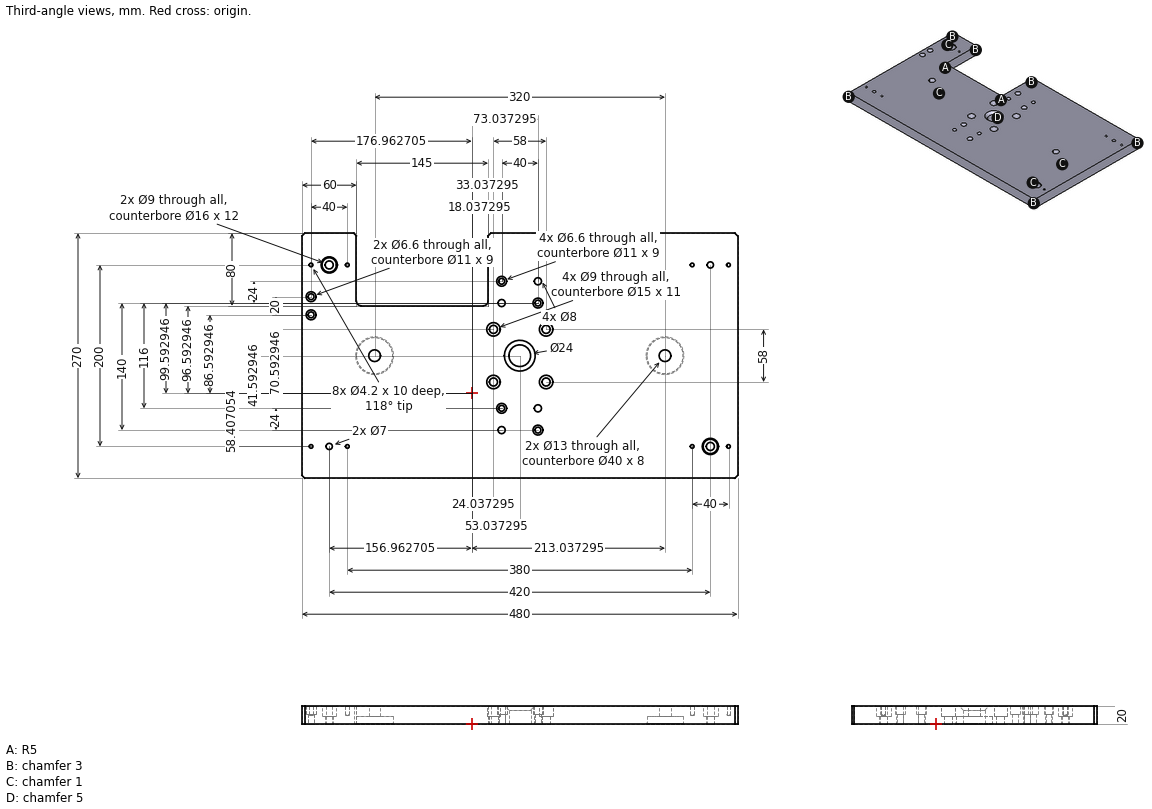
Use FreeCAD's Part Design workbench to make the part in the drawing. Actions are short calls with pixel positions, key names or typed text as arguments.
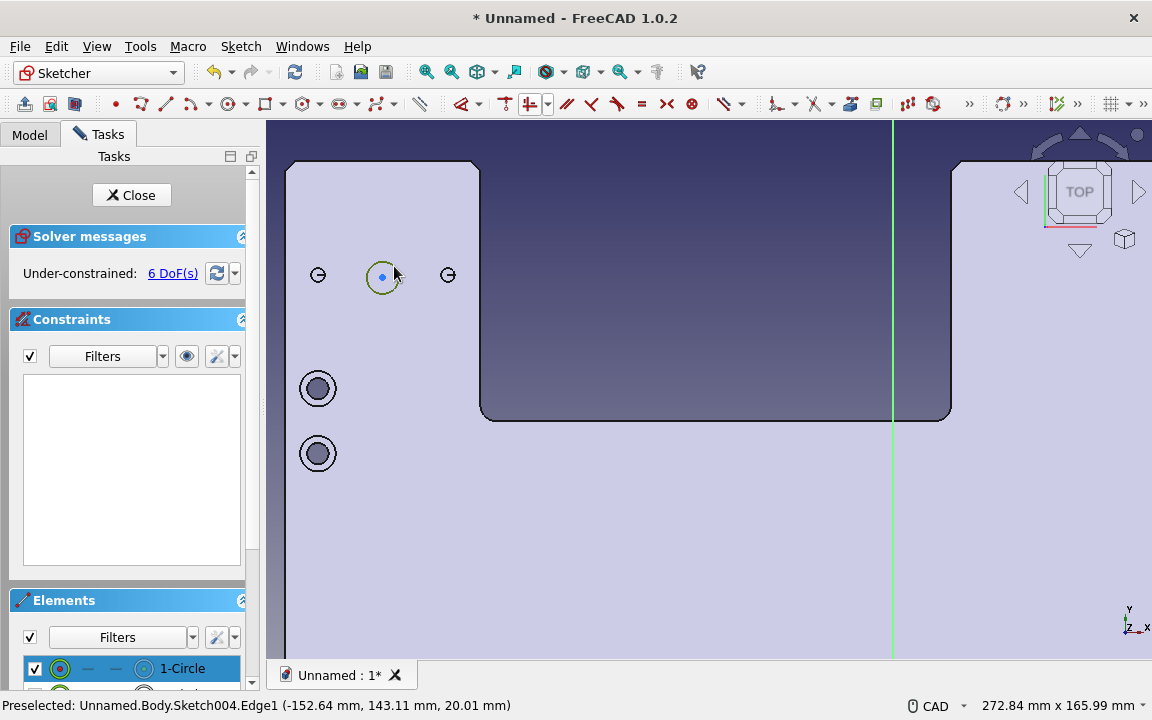
scroll(394, 267, down, 5)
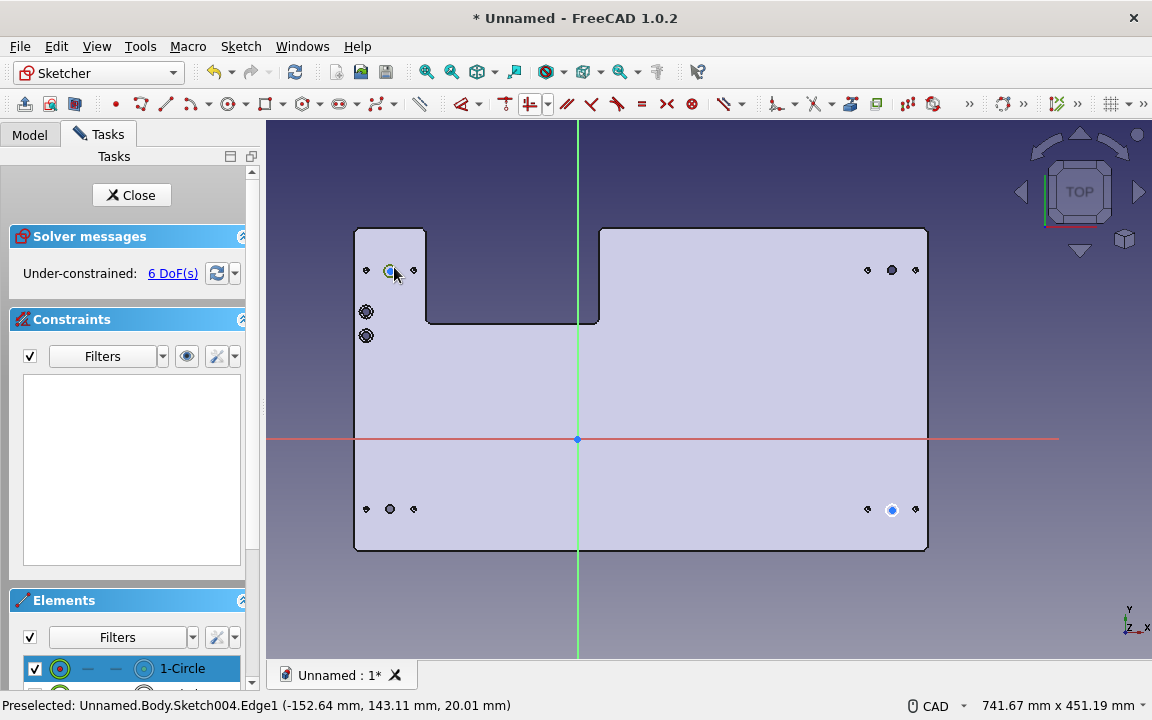
scroll(896, 506, up, 5)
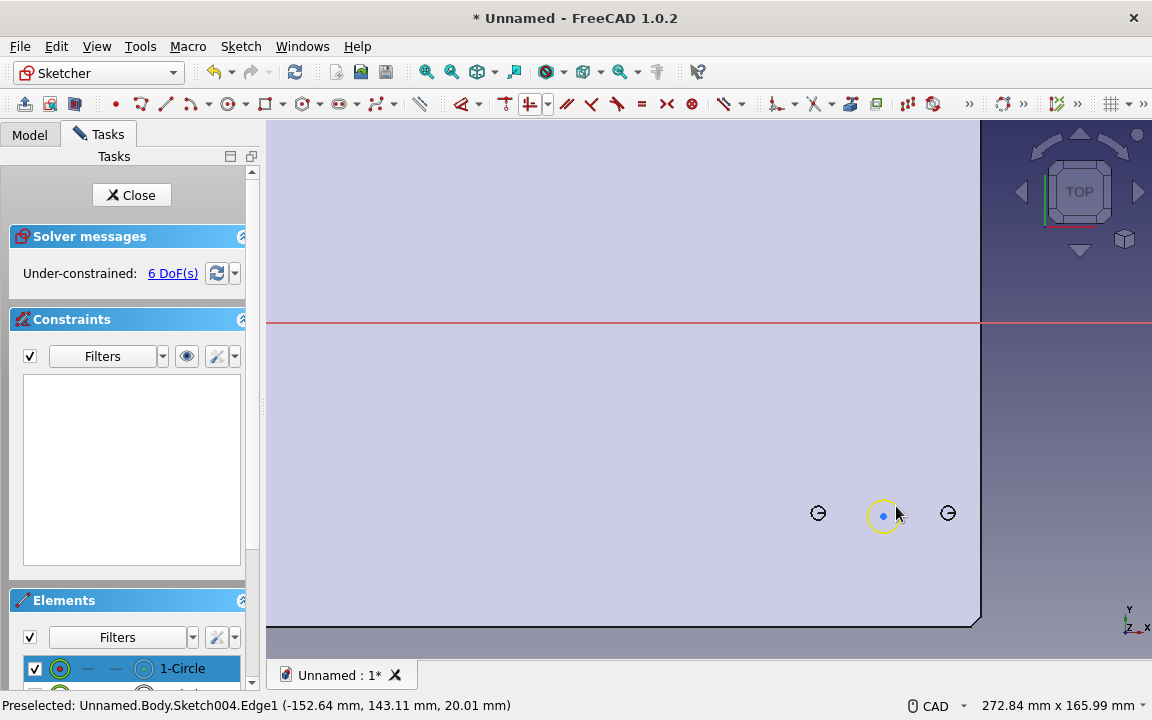
click(895, 505)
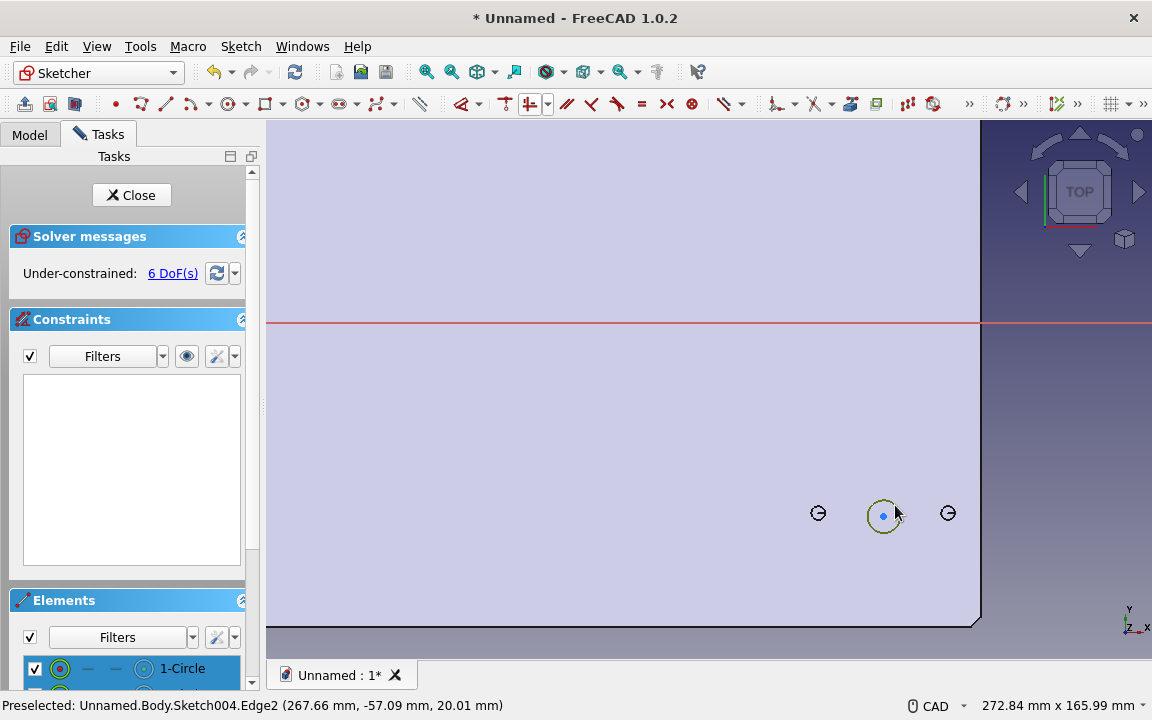
key(e)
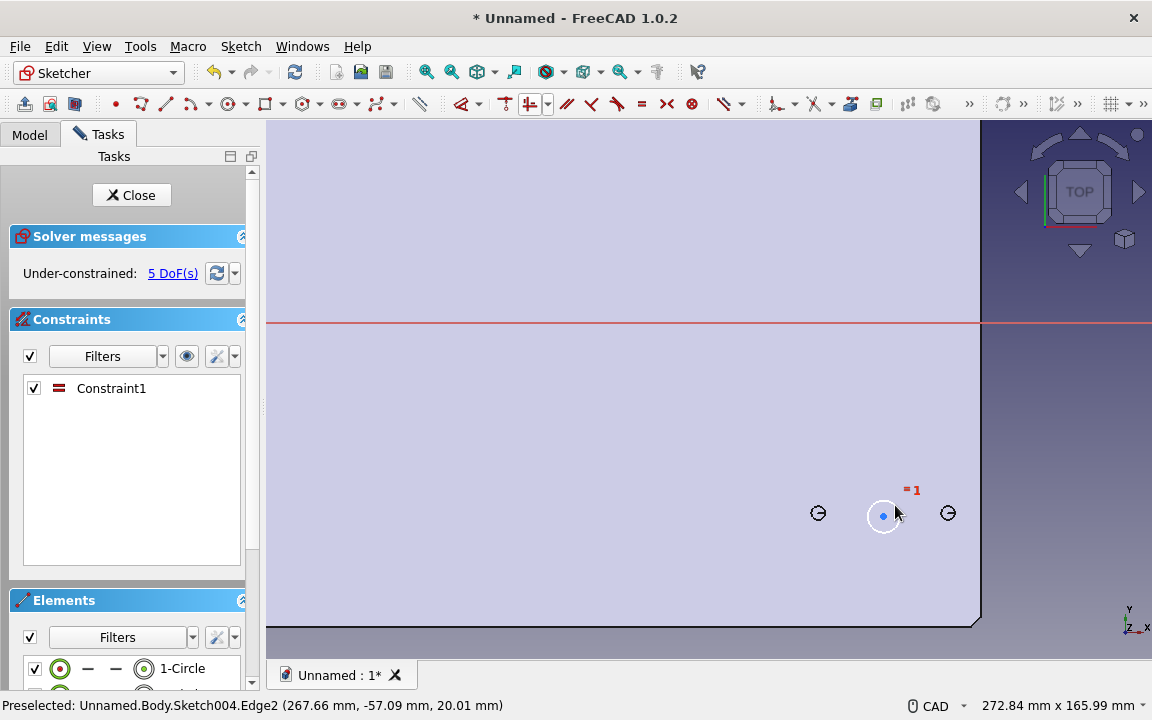
key(d)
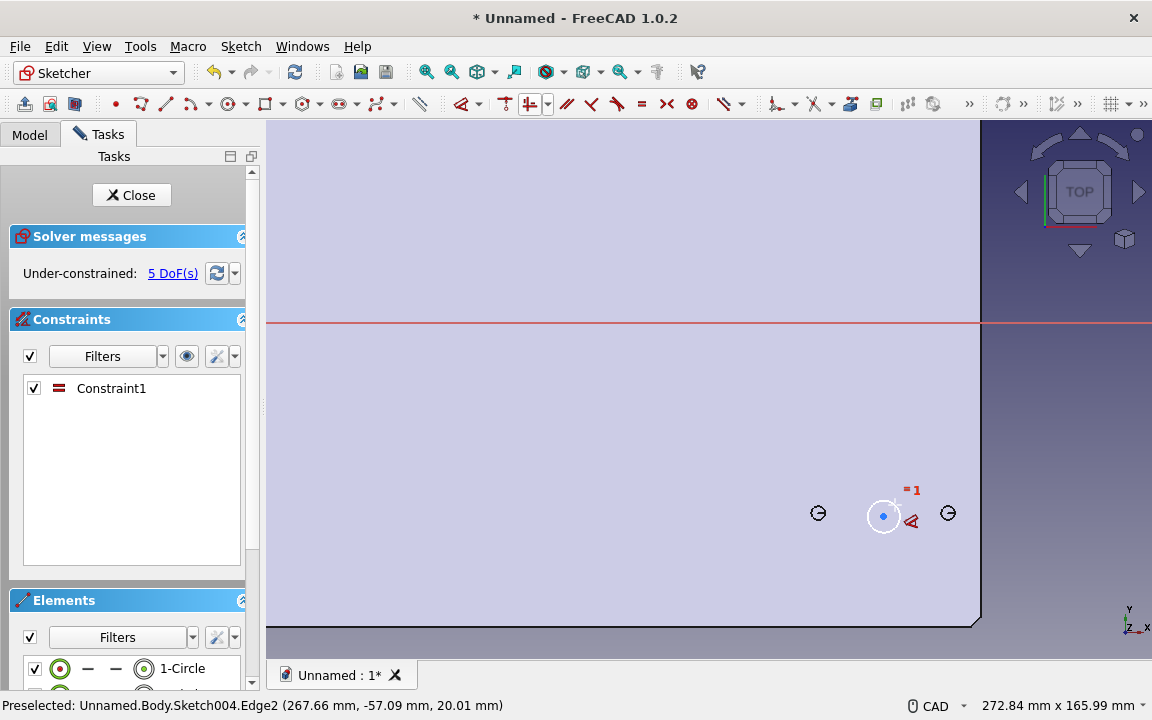
scroll(896, 507, down, 5)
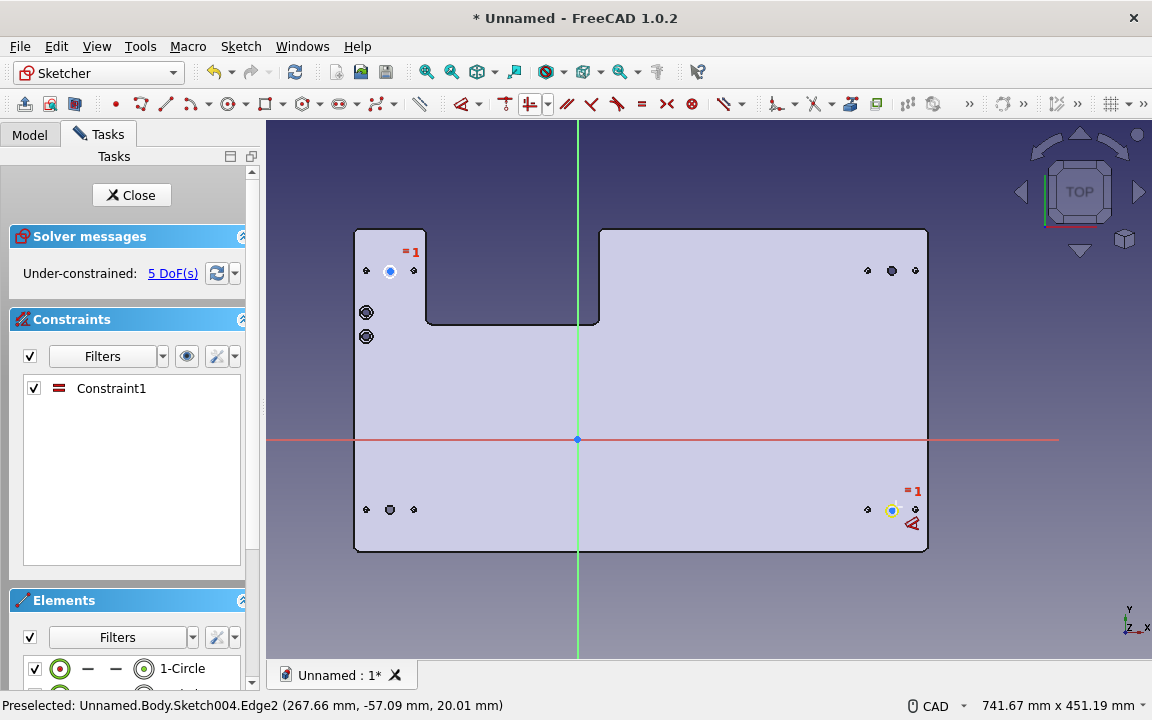
scroll(394, 268, up, 7)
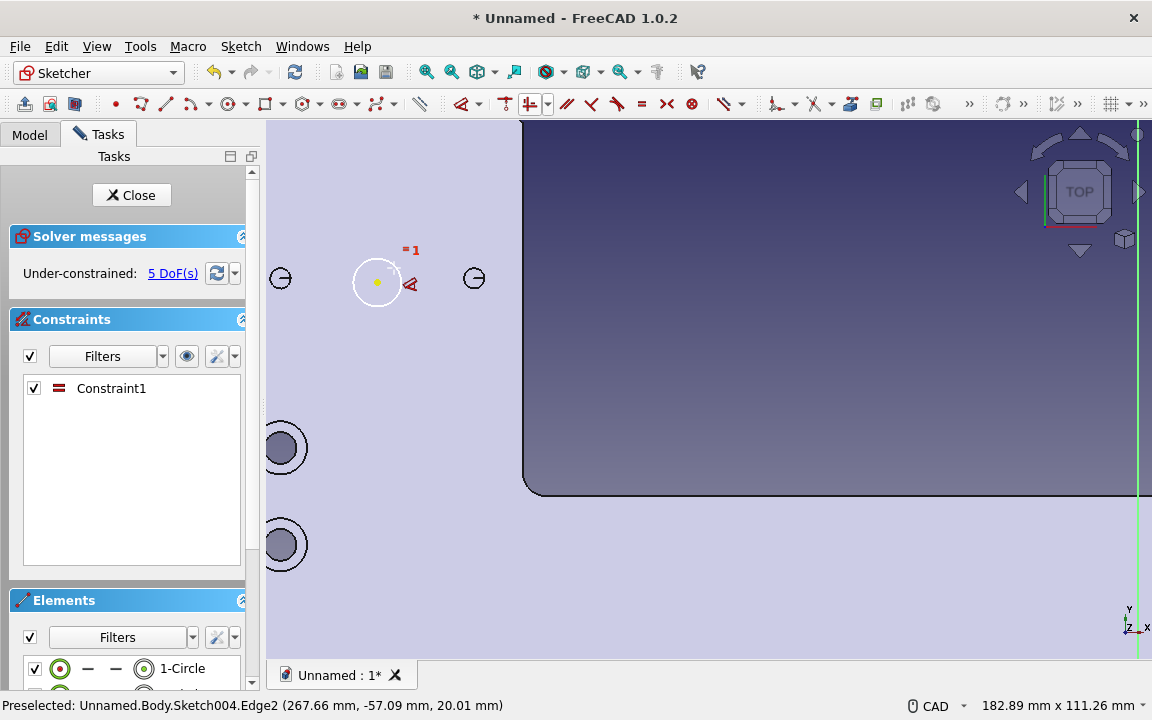
click(394, 266)
click(417, 243)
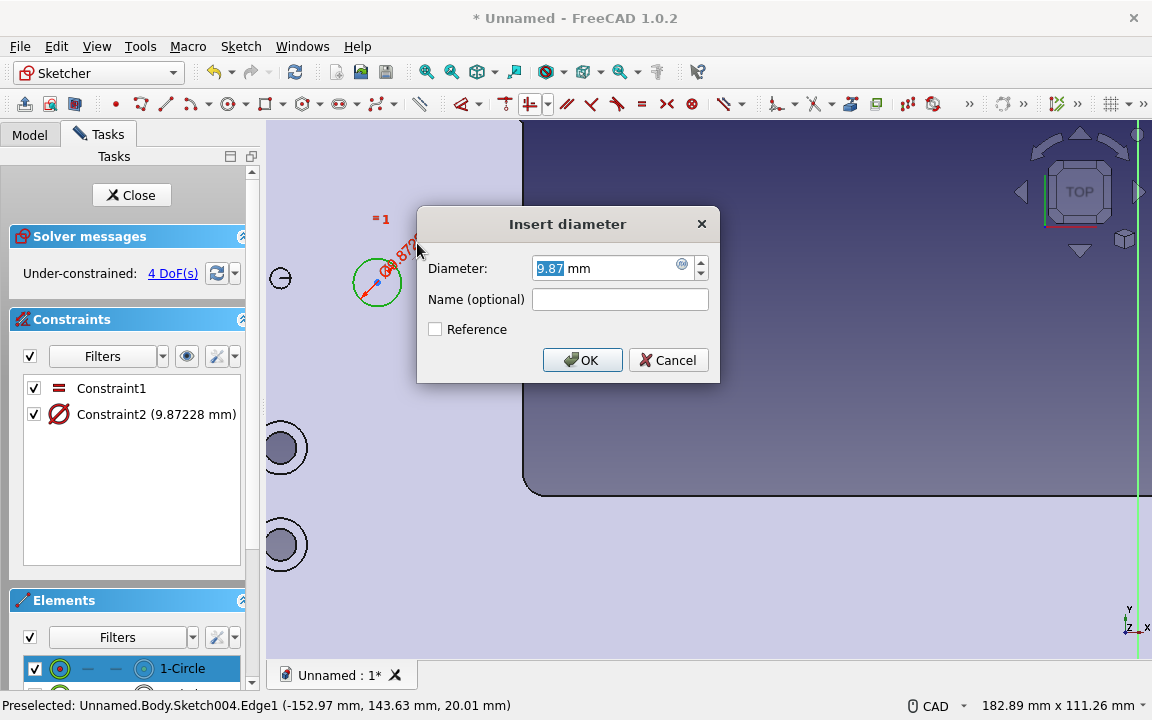
text(9)
key(Return)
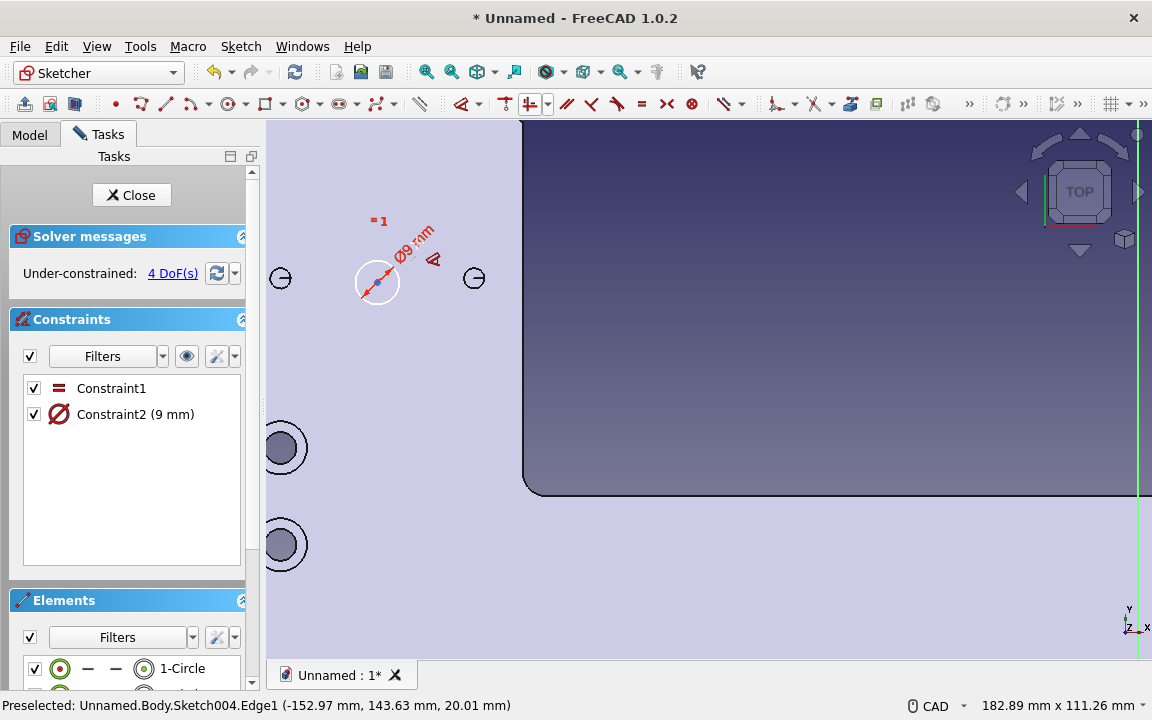
scroll(394, 267, down, 7)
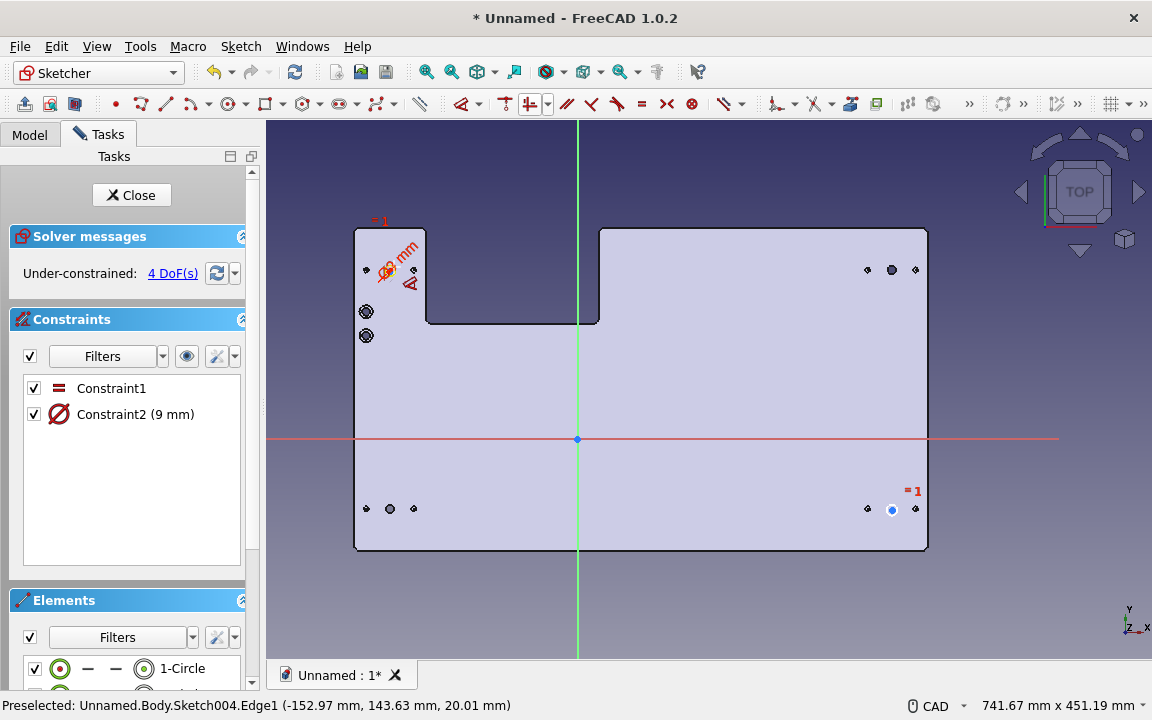
click(390, 271)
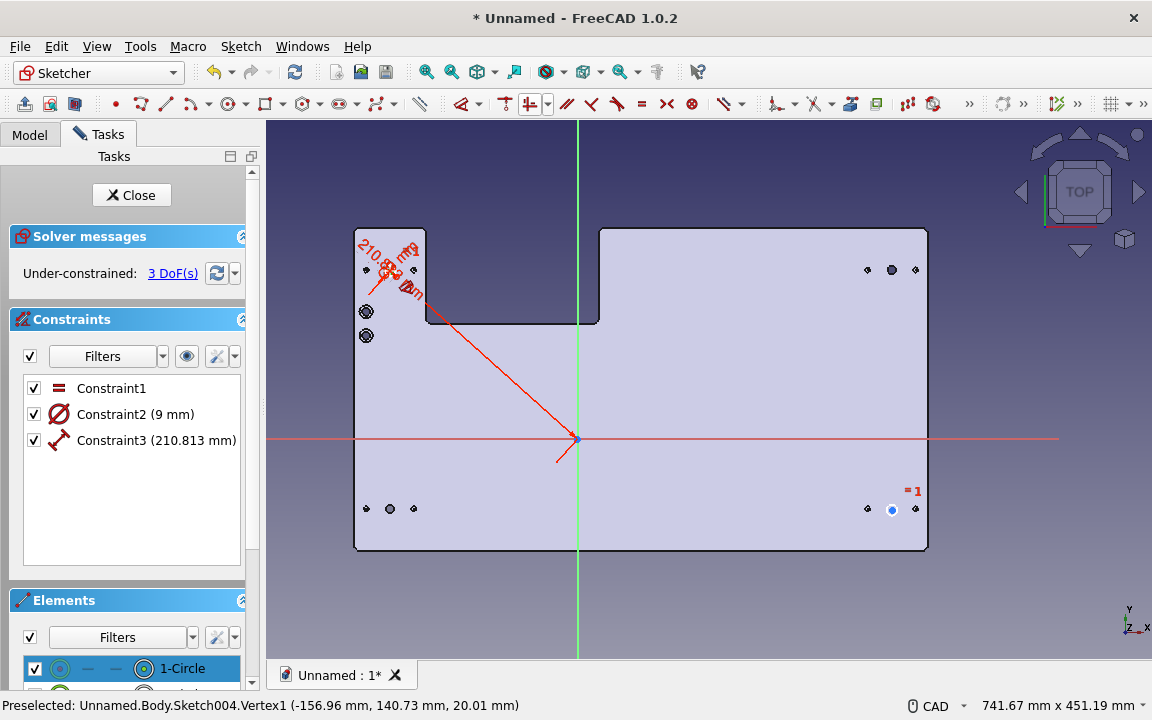
click(892, 510)
click(641, 544)